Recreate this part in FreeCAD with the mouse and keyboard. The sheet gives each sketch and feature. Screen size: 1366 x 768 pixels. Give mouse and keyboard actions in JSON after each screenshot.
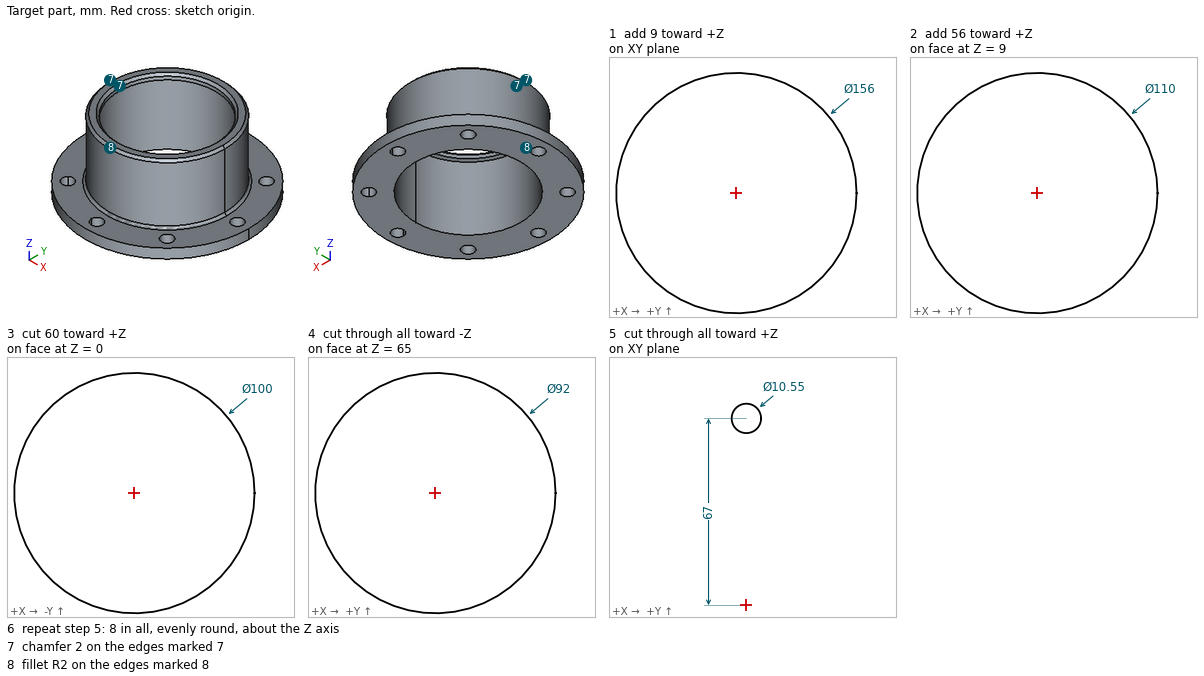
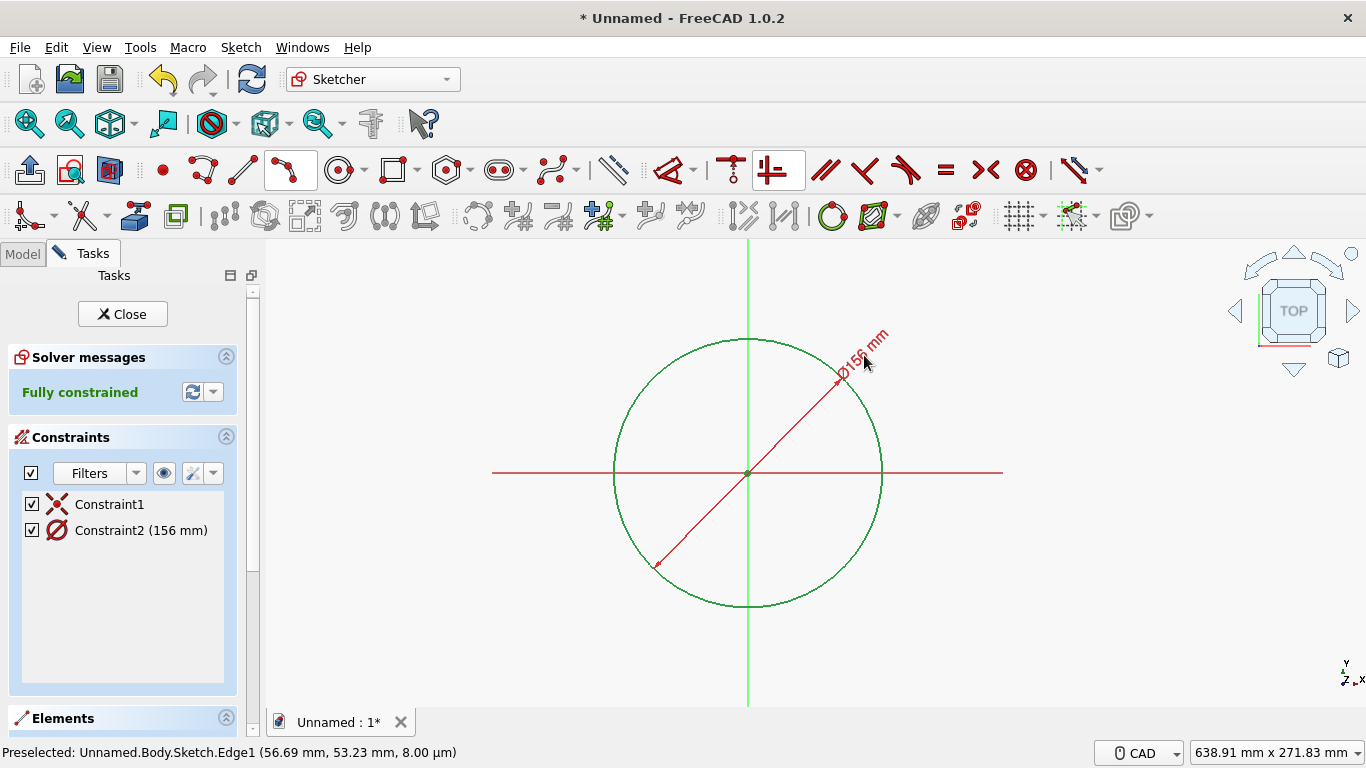
{"action": "left_click", "coordinate": [123, 314]}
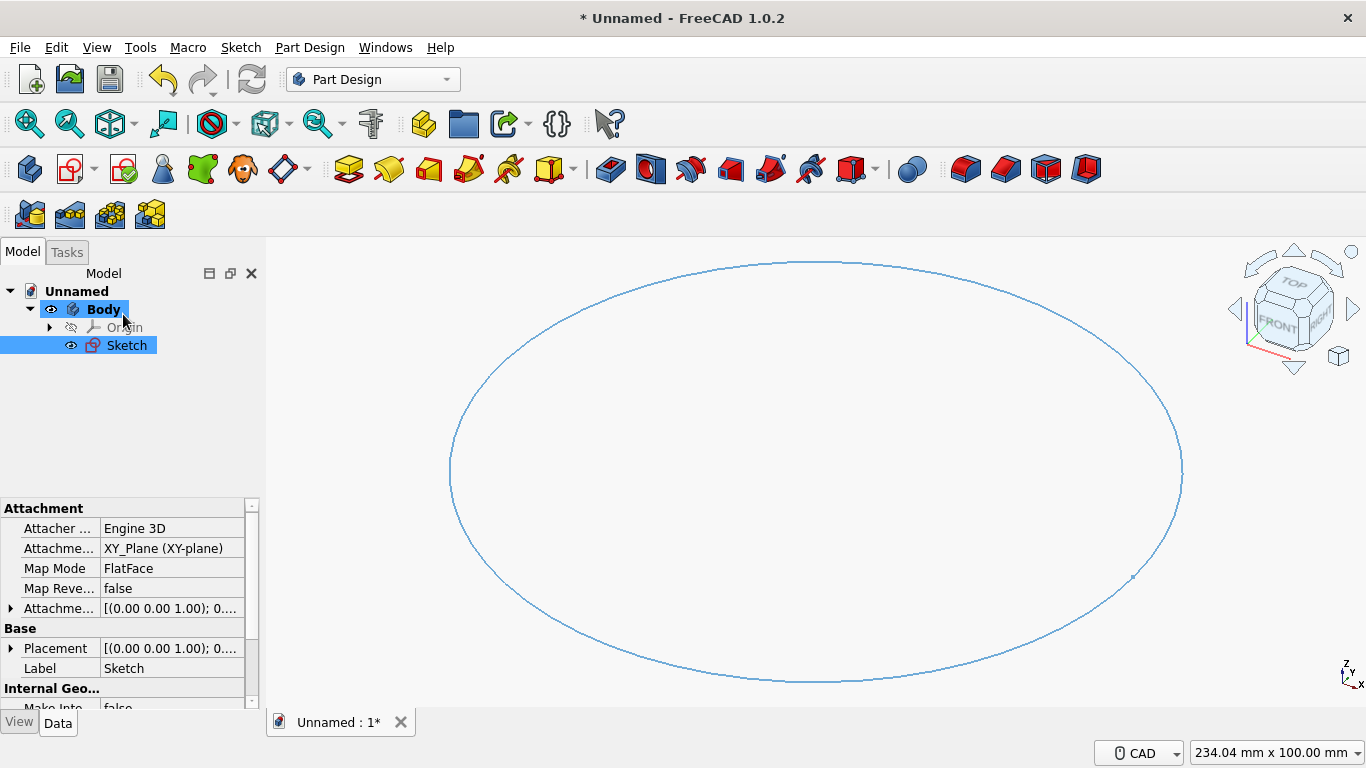
{"action": "left_click", "coordinate": [350, 170]}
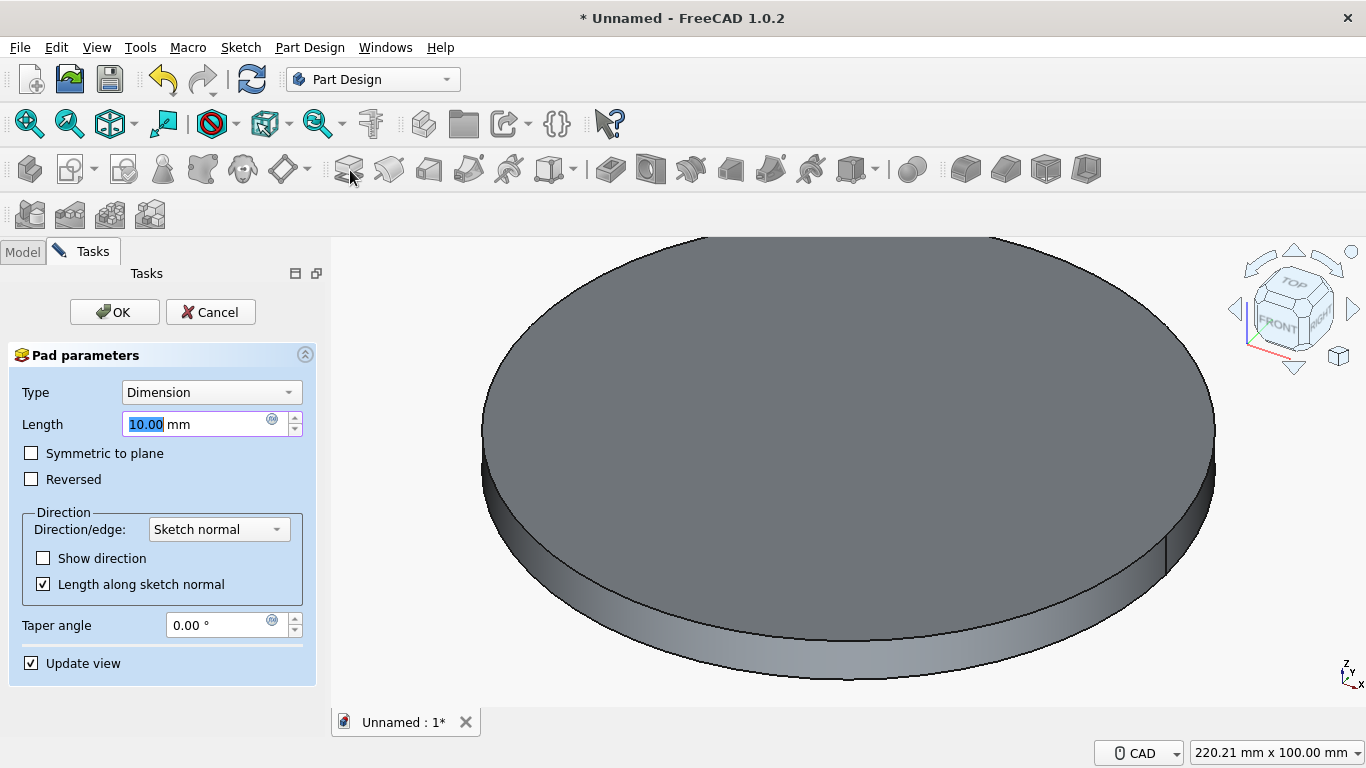
{"action": "type", "text": "9"}
{"action": "key", "text": "Tab"}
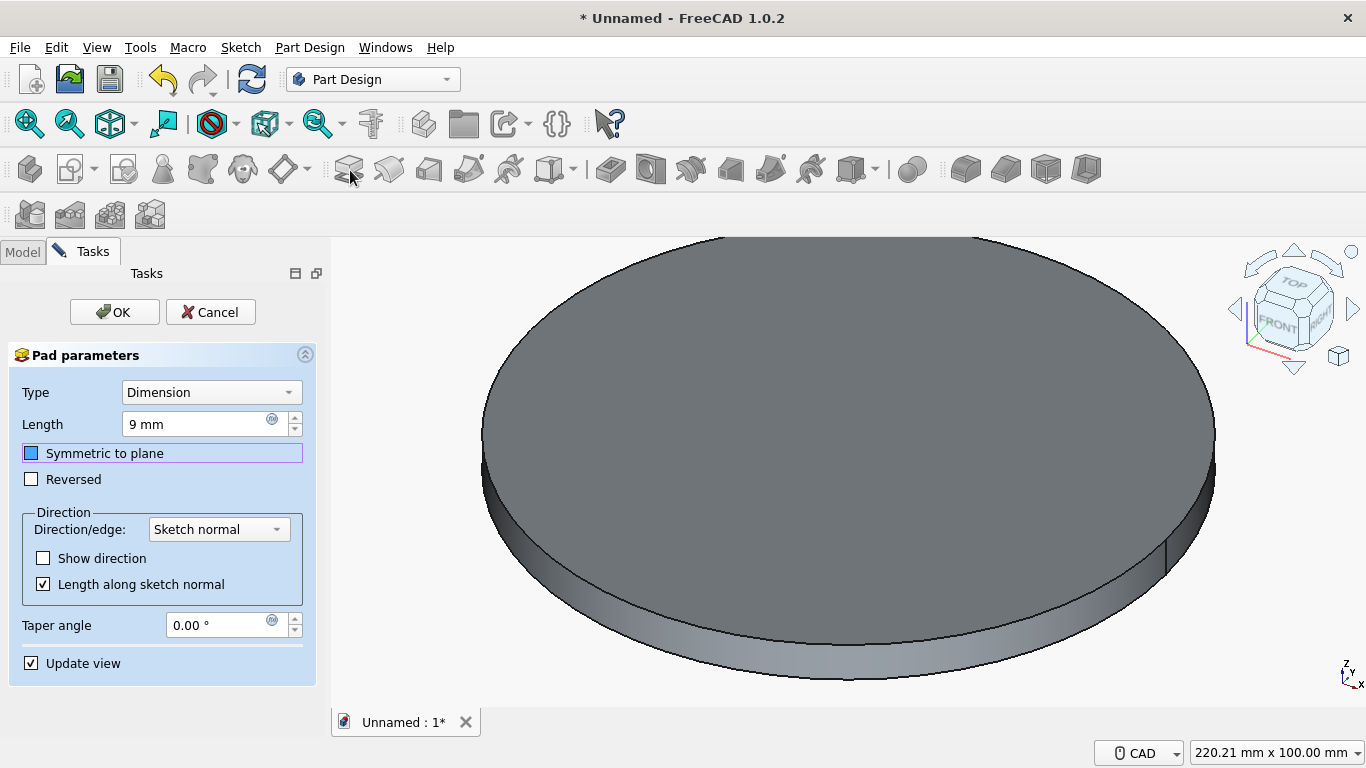
{"action": "left_click", "coordinate": [115, 312]}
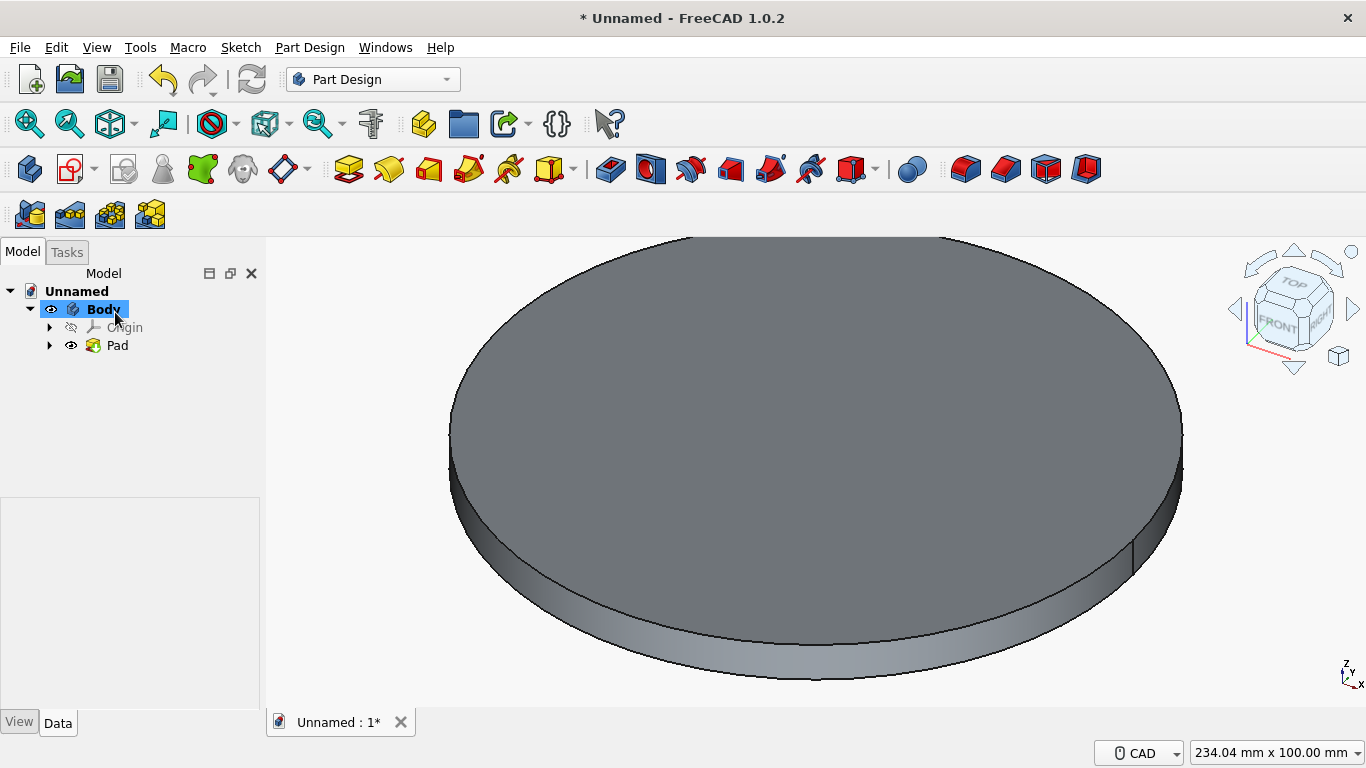
{"action": "left_click", "coordinate": [30, 124]}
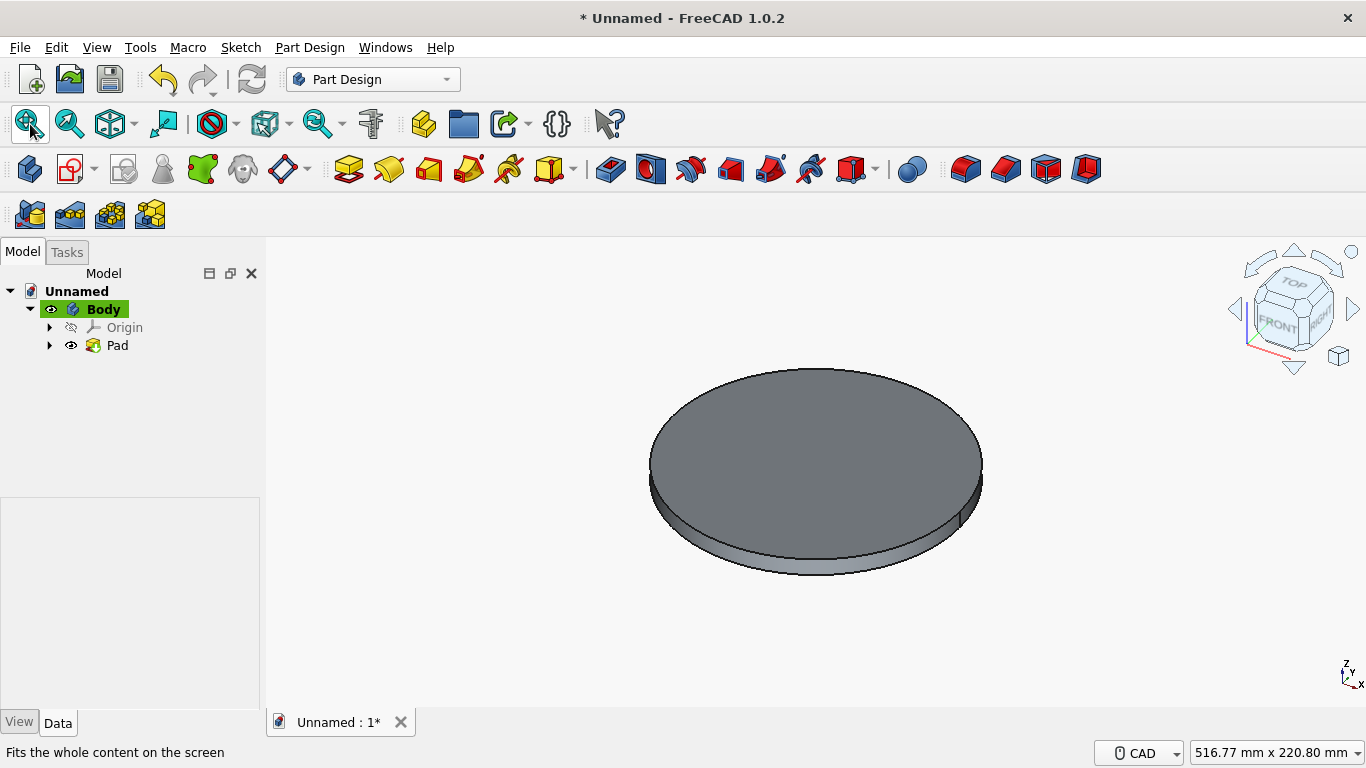
{"action": "left_click", "coordinate": [816, 463]}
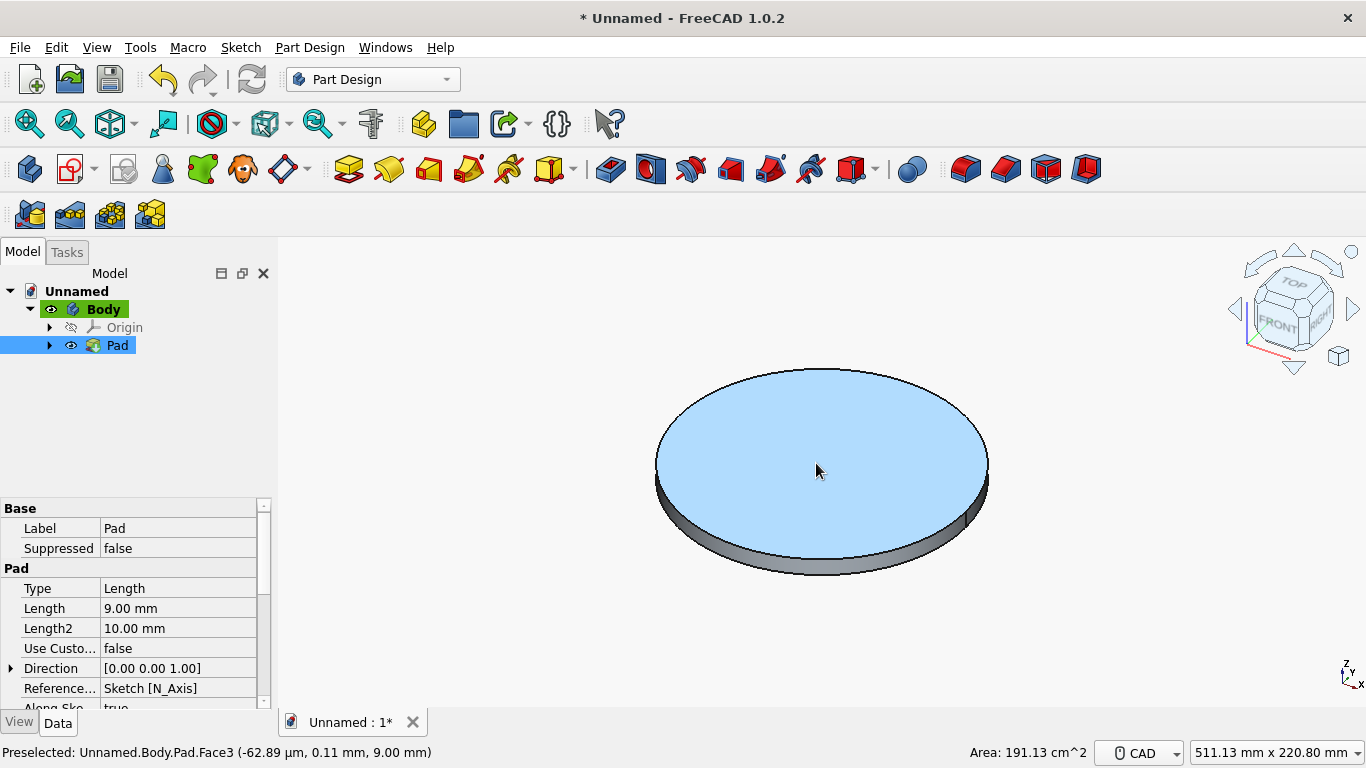
{"action": "left_click", "coordinate": [70, 170]}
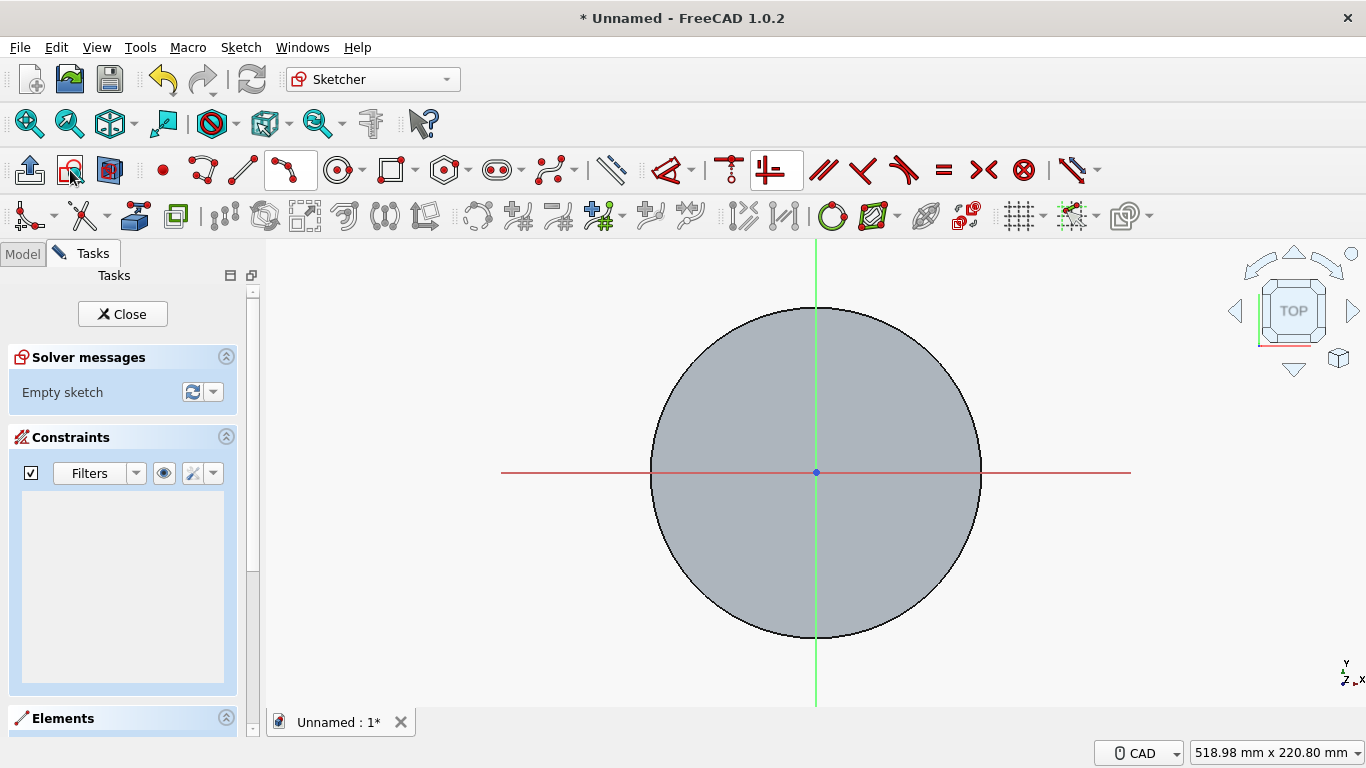
{"action": "left_click", "coordinate": [338, 170]}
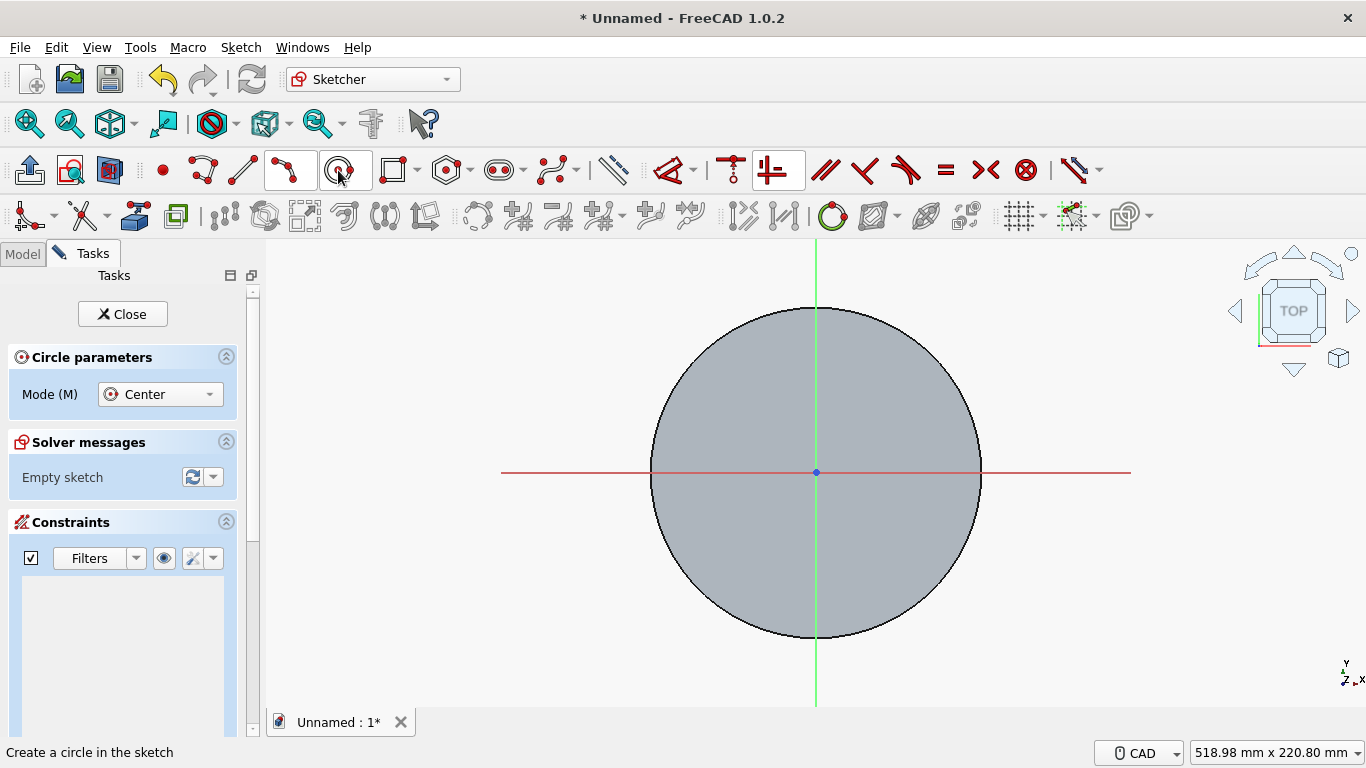
{"action": "left_click", "coordinate": [816, 473]}
{"action": "left_click", "coordinate": [898, 391]}
{"action": "key", "text": "Escape"}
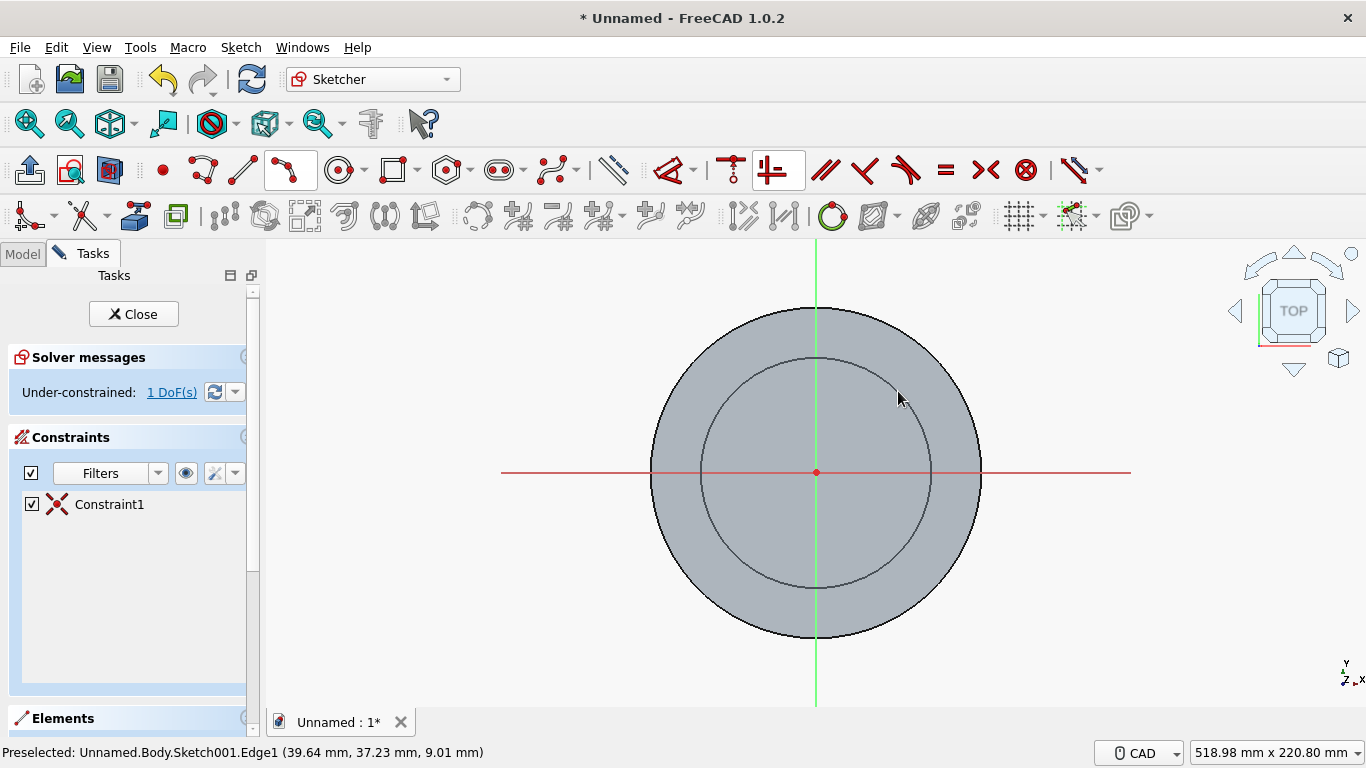
{"action": "left_click", "coordinate": [668, 170]}